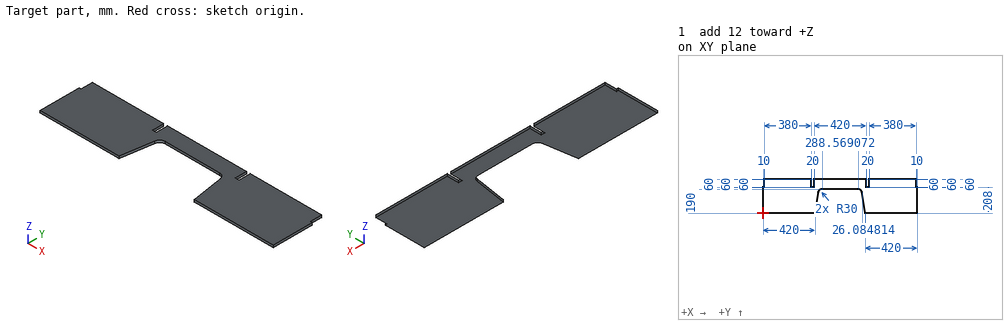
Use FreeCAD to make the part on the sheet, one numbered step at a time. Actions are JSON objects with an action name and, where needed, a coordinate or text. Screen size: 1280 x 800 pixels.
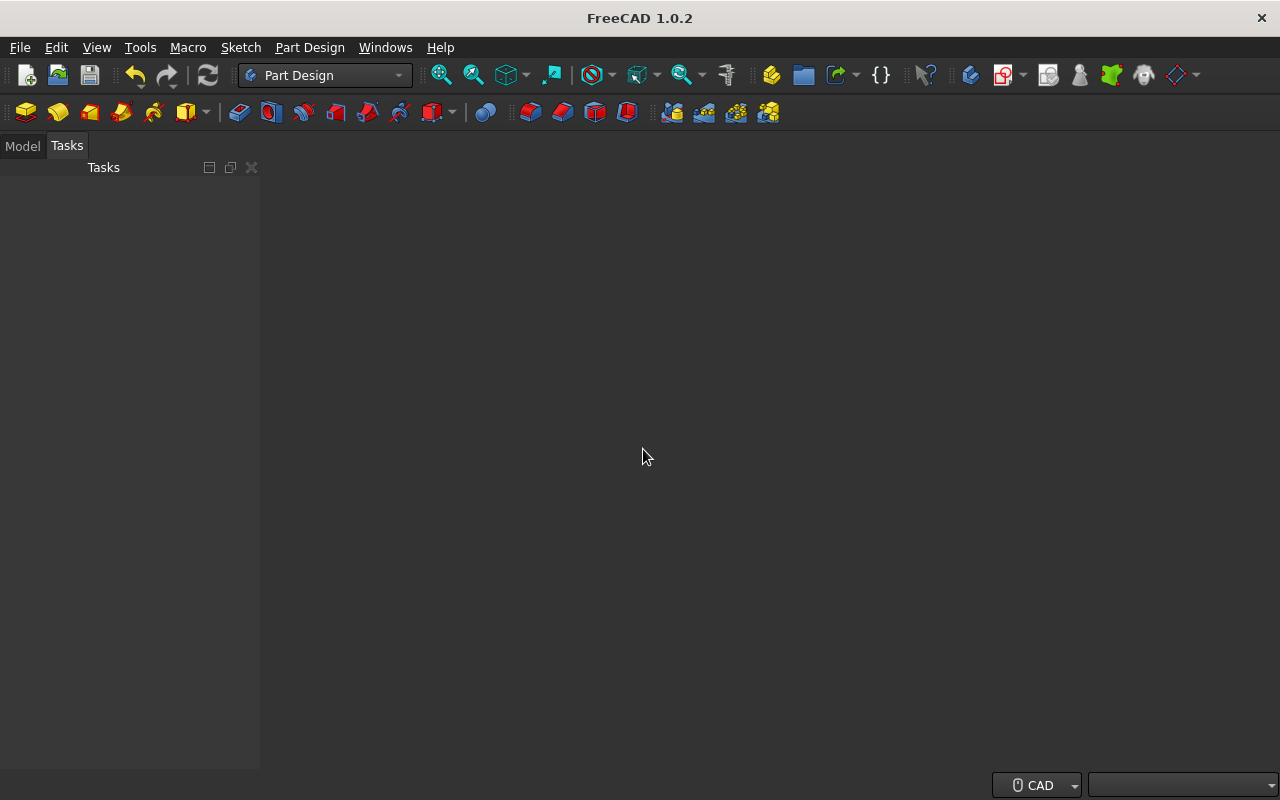
{"action": "key", "text": "ctrl+n"}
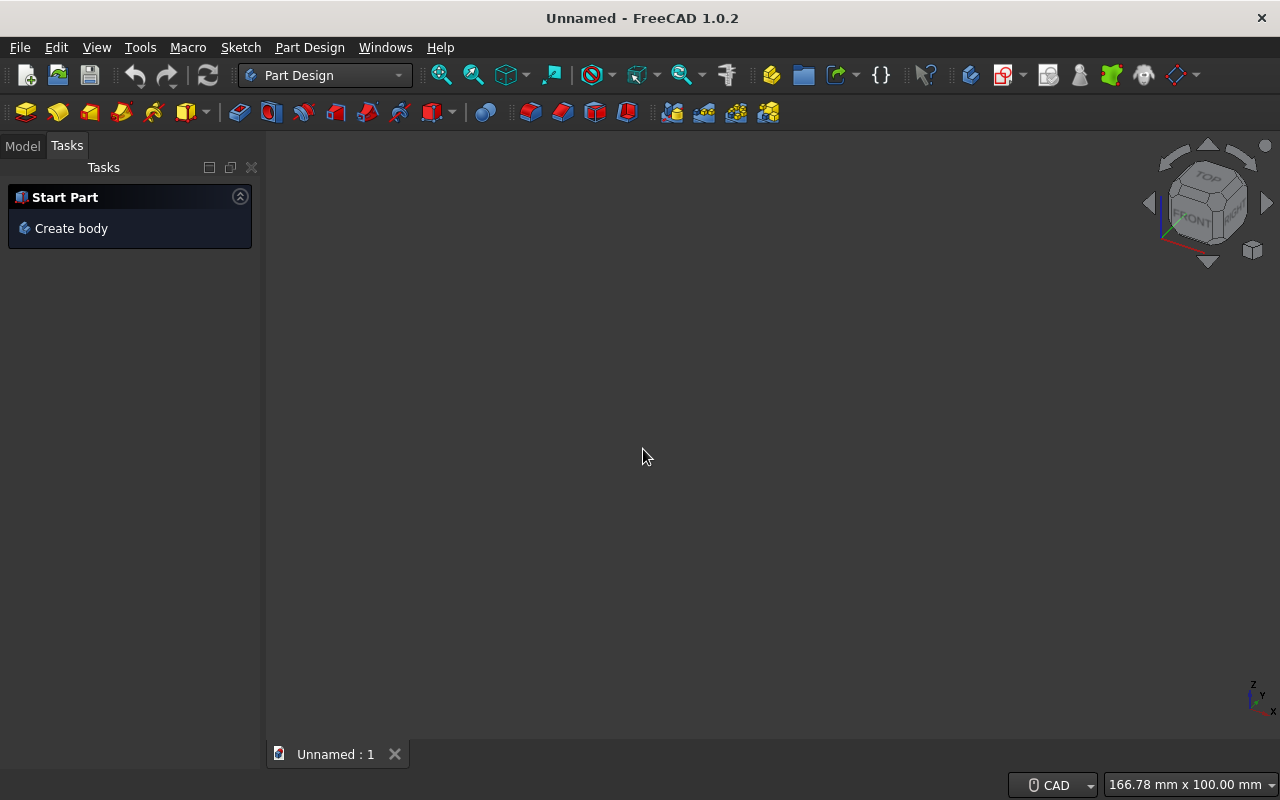
{"action": "left_click", "coordinate": [1004, 76]}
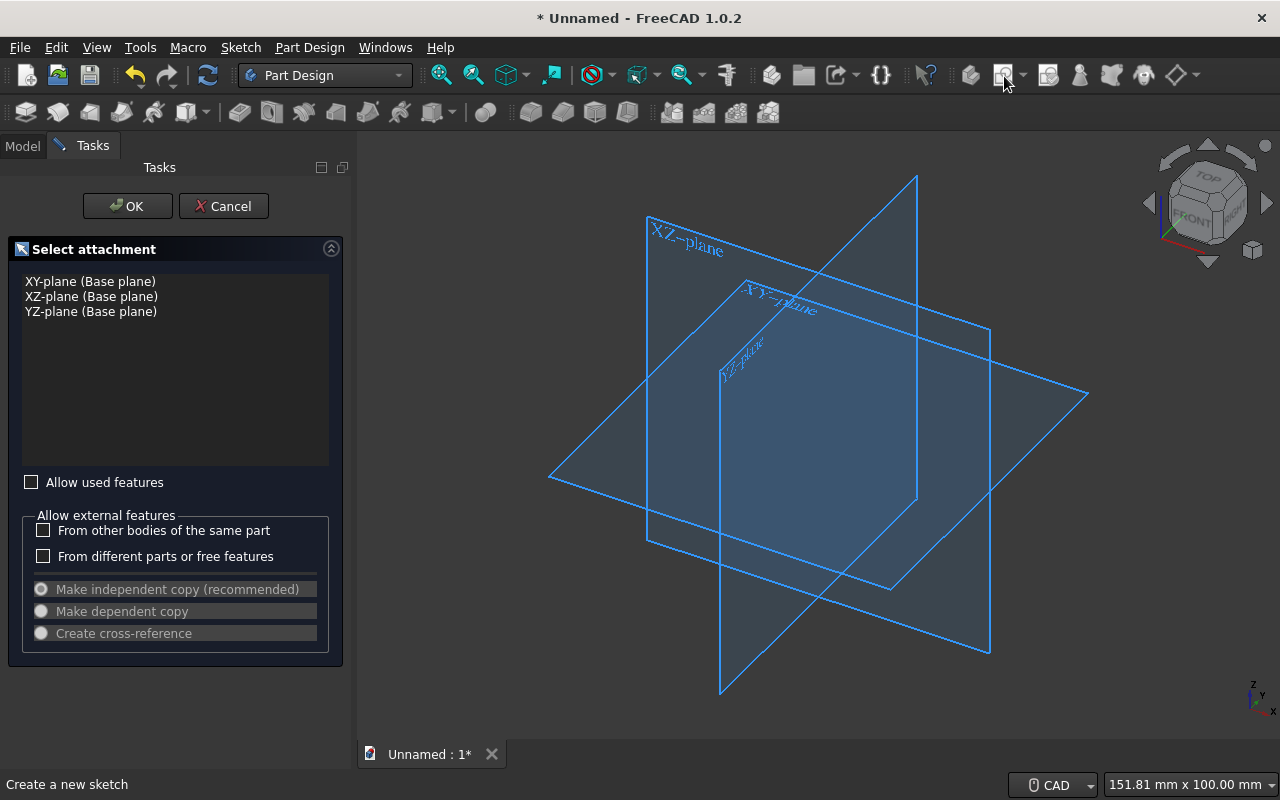
{"action": "left_click", "coordinate": [82, 282]}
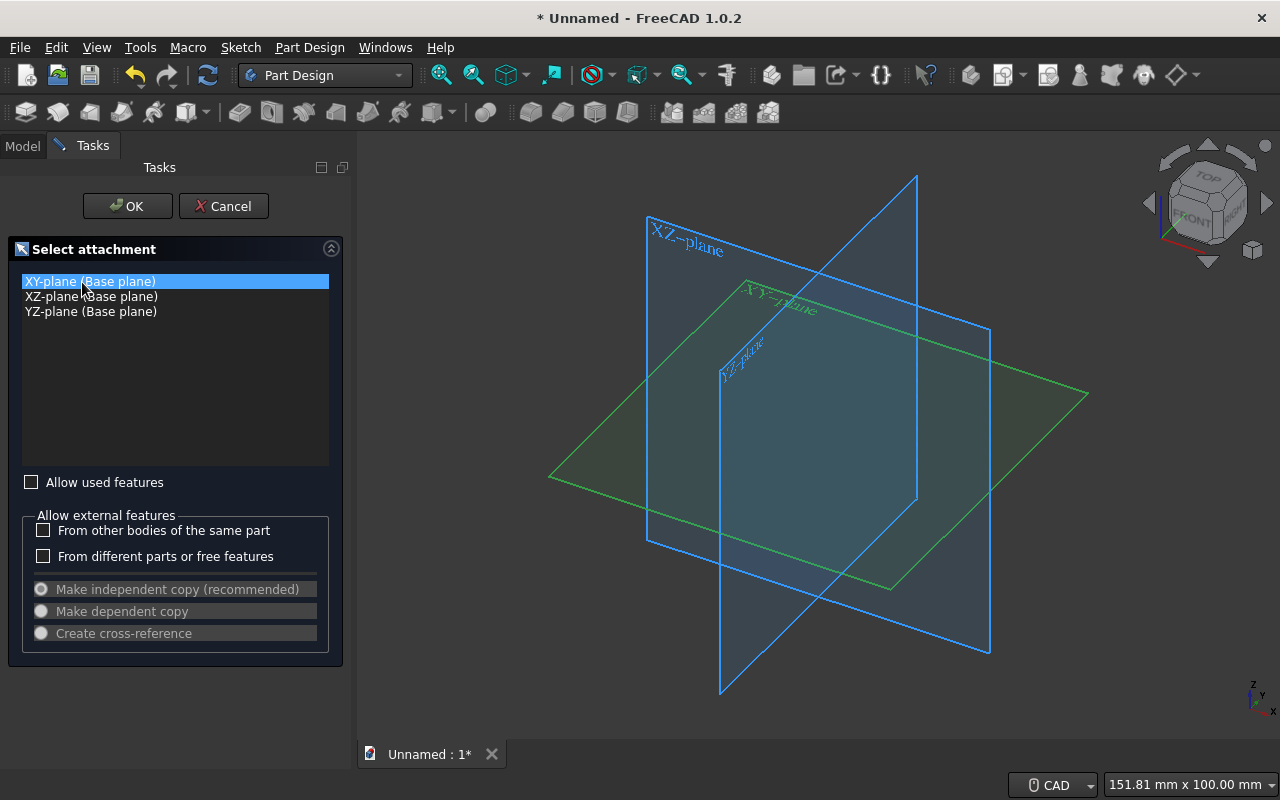
{"action": "left_click", "coordinate": [128, 206]}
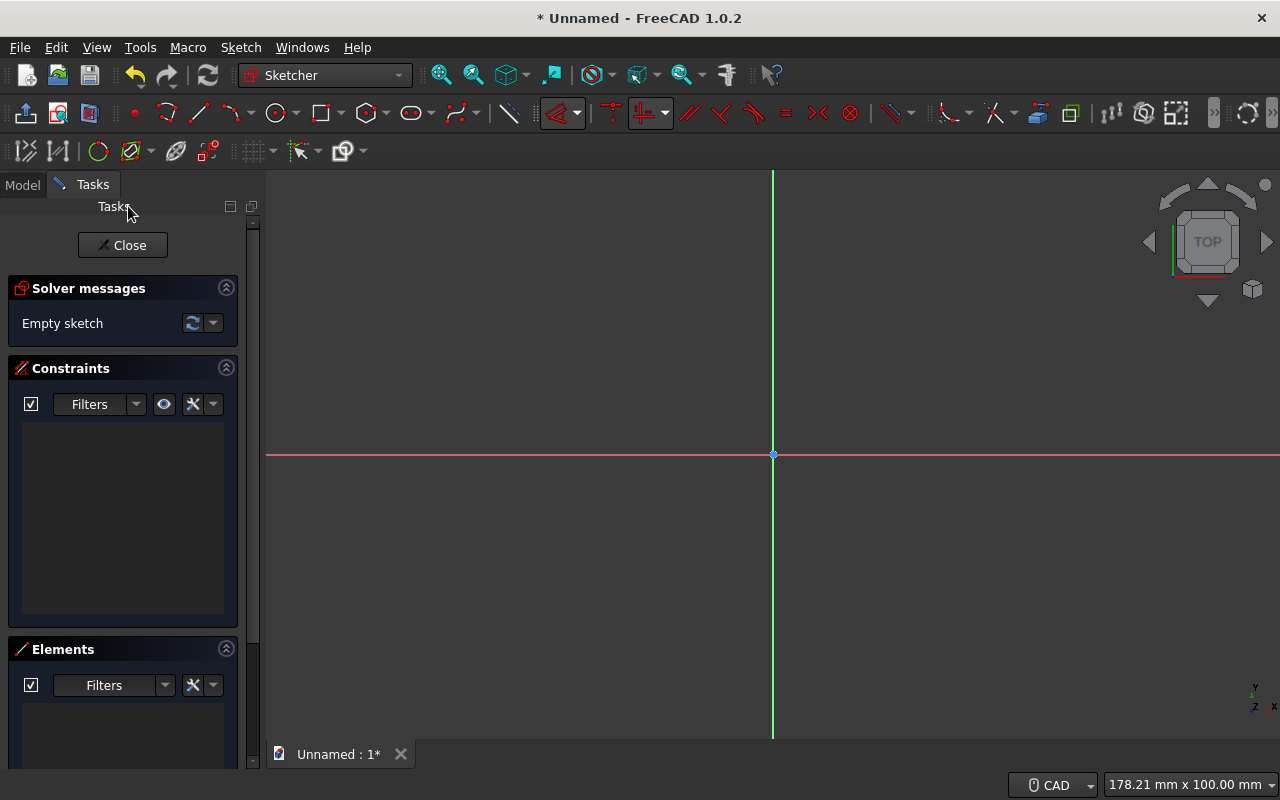
{"action": "scroll", "coordinate": [346, 531], "scroll_direction": "down", "scroll_amount": 12}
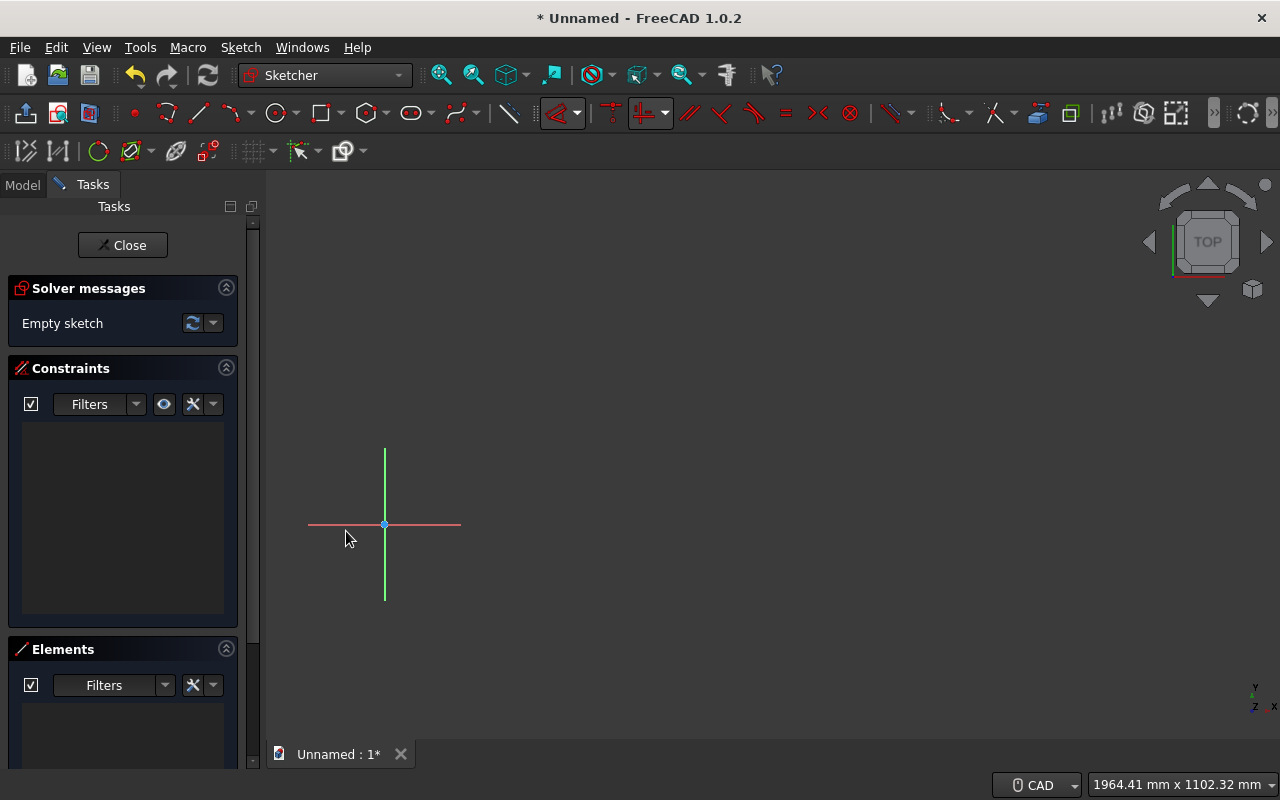
{"action": "left_click", "coordinate": [200, 114]}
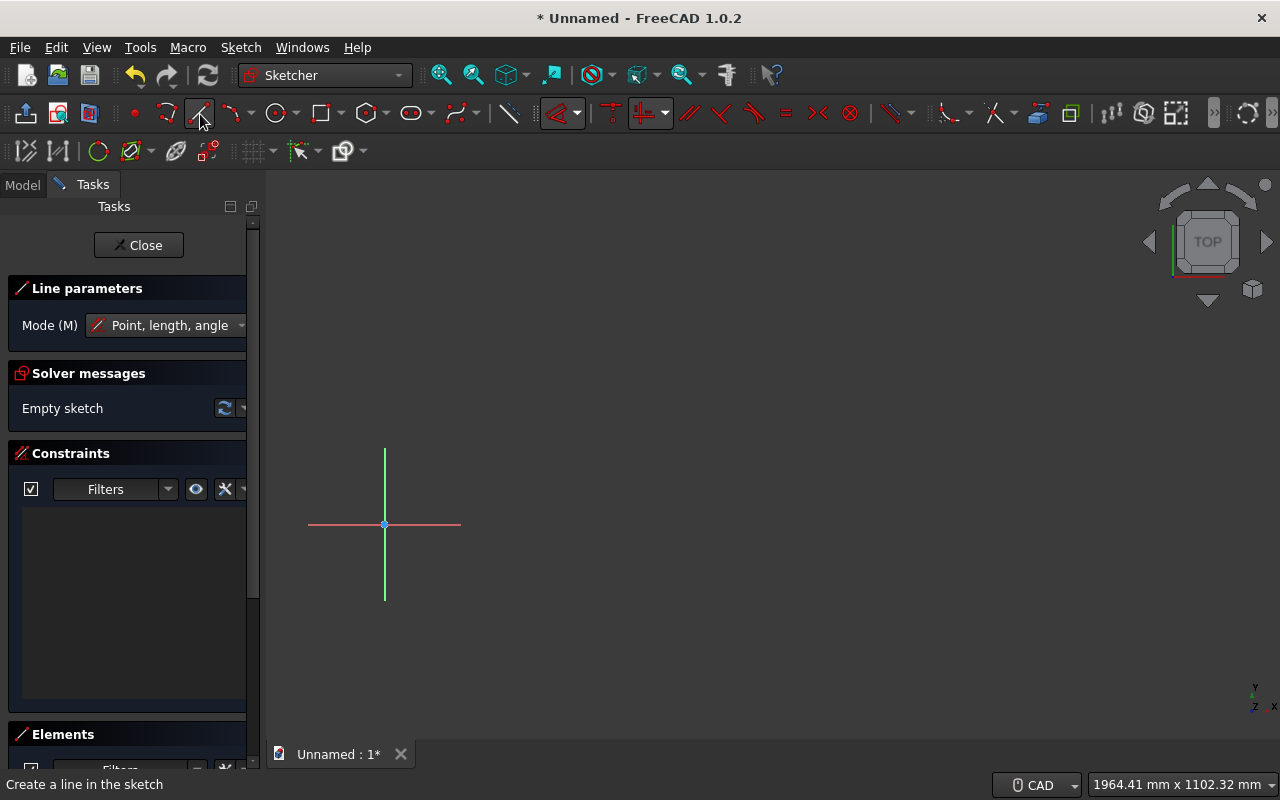
{"action": "left_click", "coordinate": [630, 427]}
{"action": "left_click", "coordinate": [779, 427]}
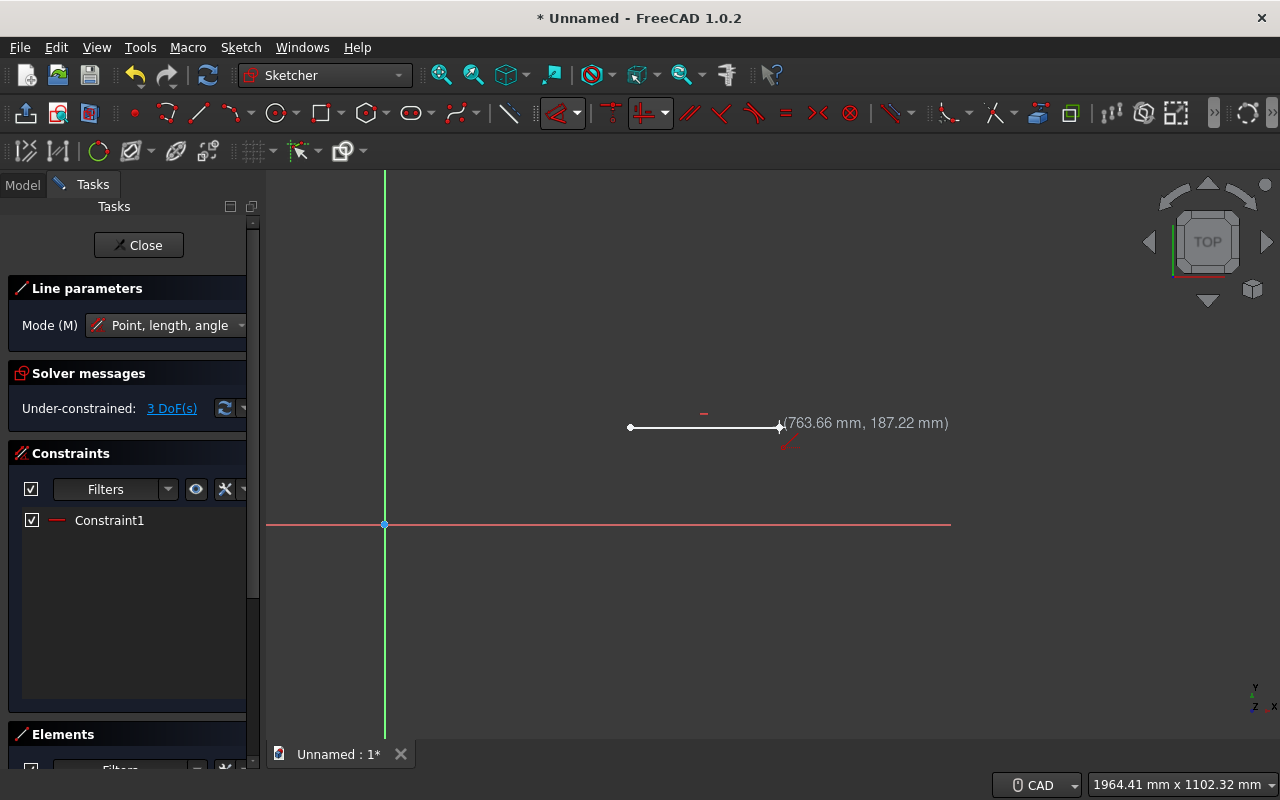
{"action": "key", "text": "g m"}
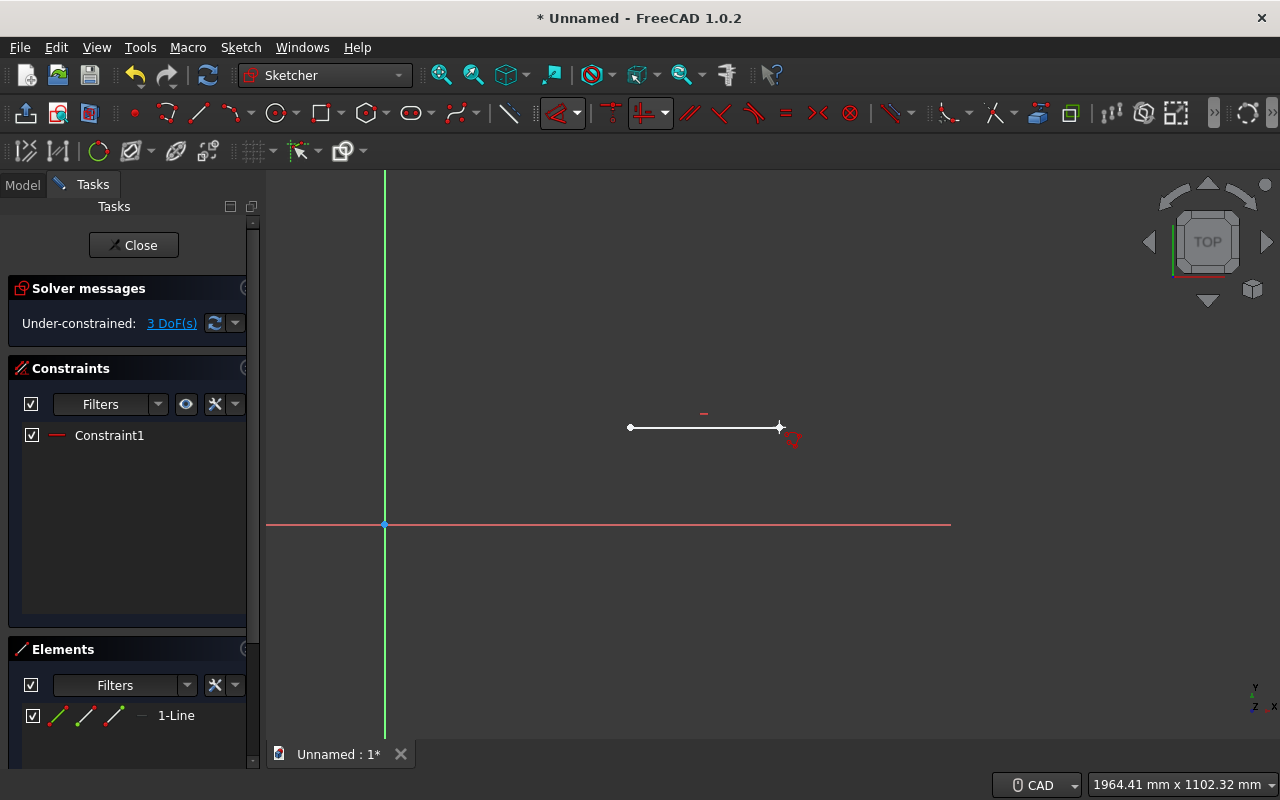
{"action": "left_click", "coordinate": [795, 440]}
{"action": "left_click", "coordinate": [808, 525]}
{"action": "left_click", "coordinate": [1025, 516]}
{"action": "left_click", "coordinate": [1025, 417]}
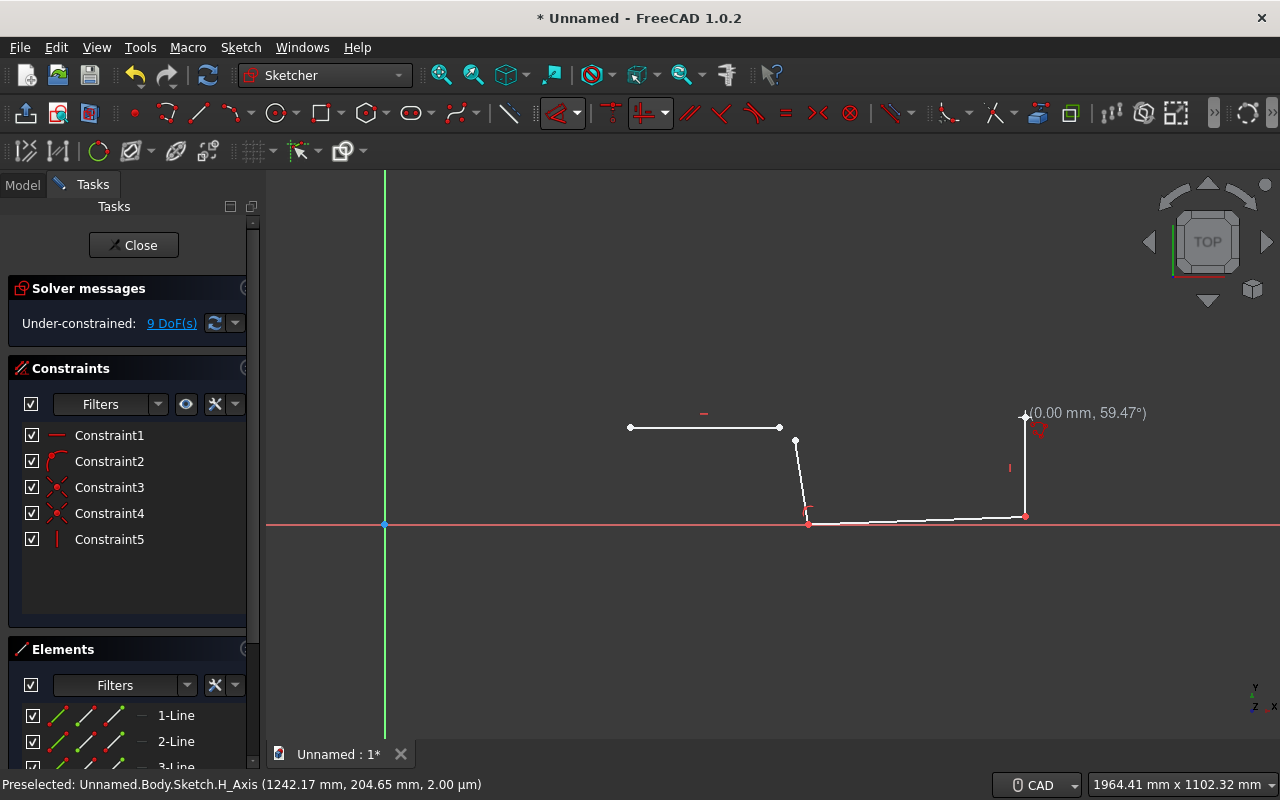
{"action": "scroll", "coordinate": [1020, 417], "scroll_direction": "up", "scroll_amount": 6}